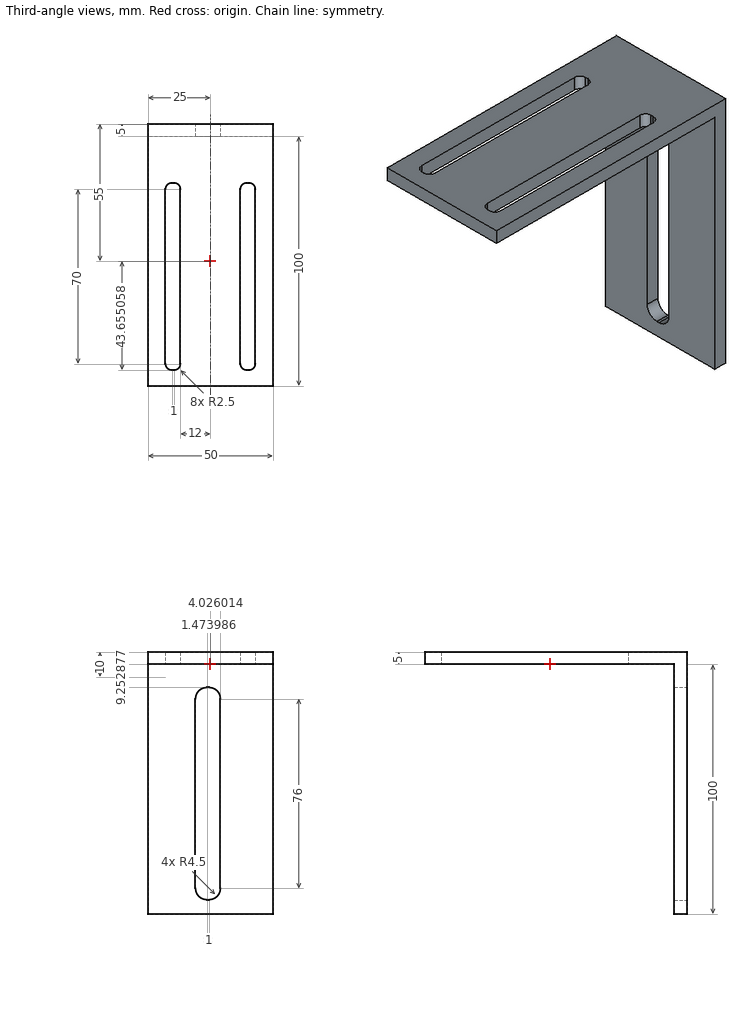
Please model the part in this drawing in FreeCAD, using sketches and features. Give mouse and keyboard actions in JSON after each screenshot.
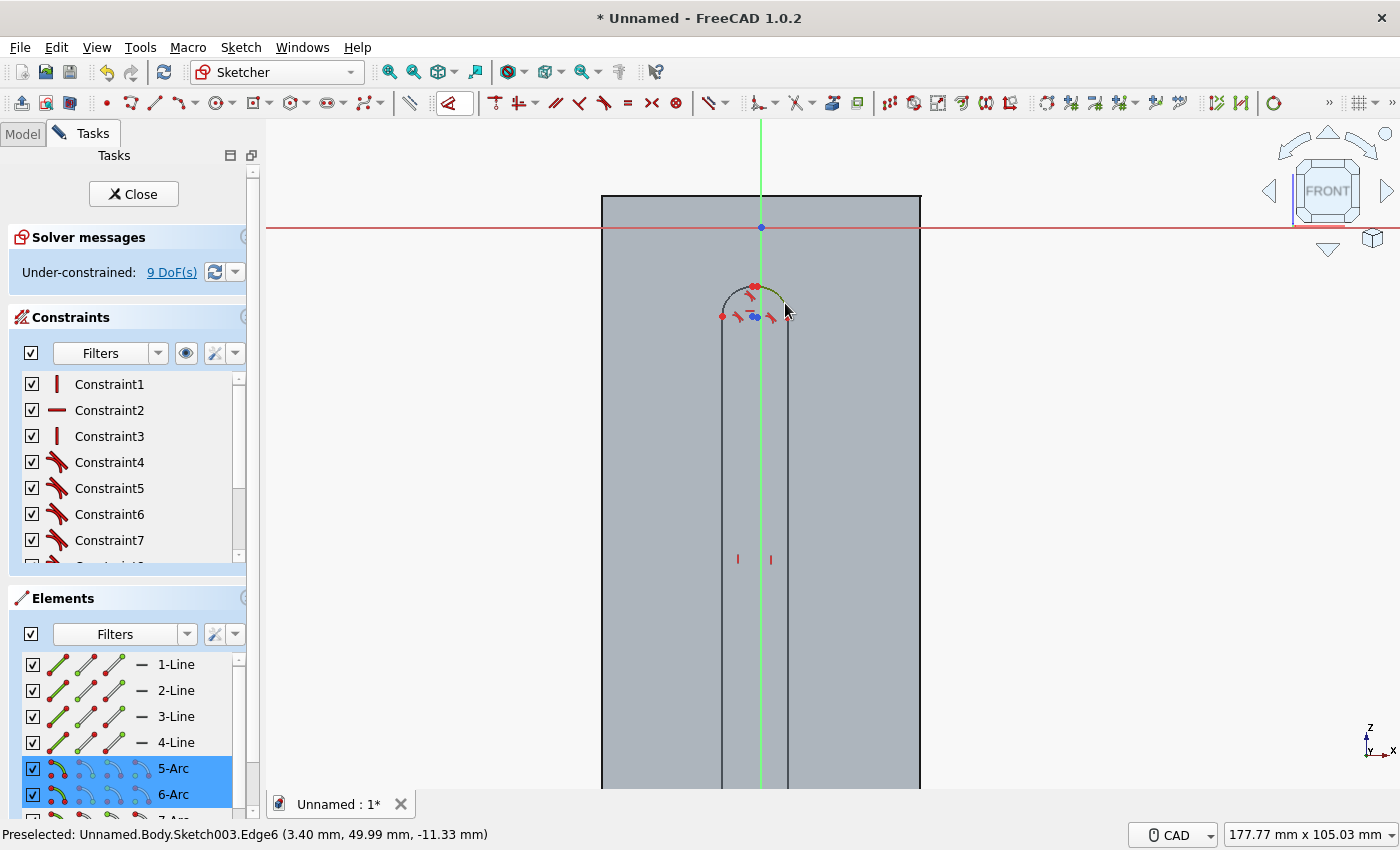
{"action": "left_click", "coordinate": [739, 290]}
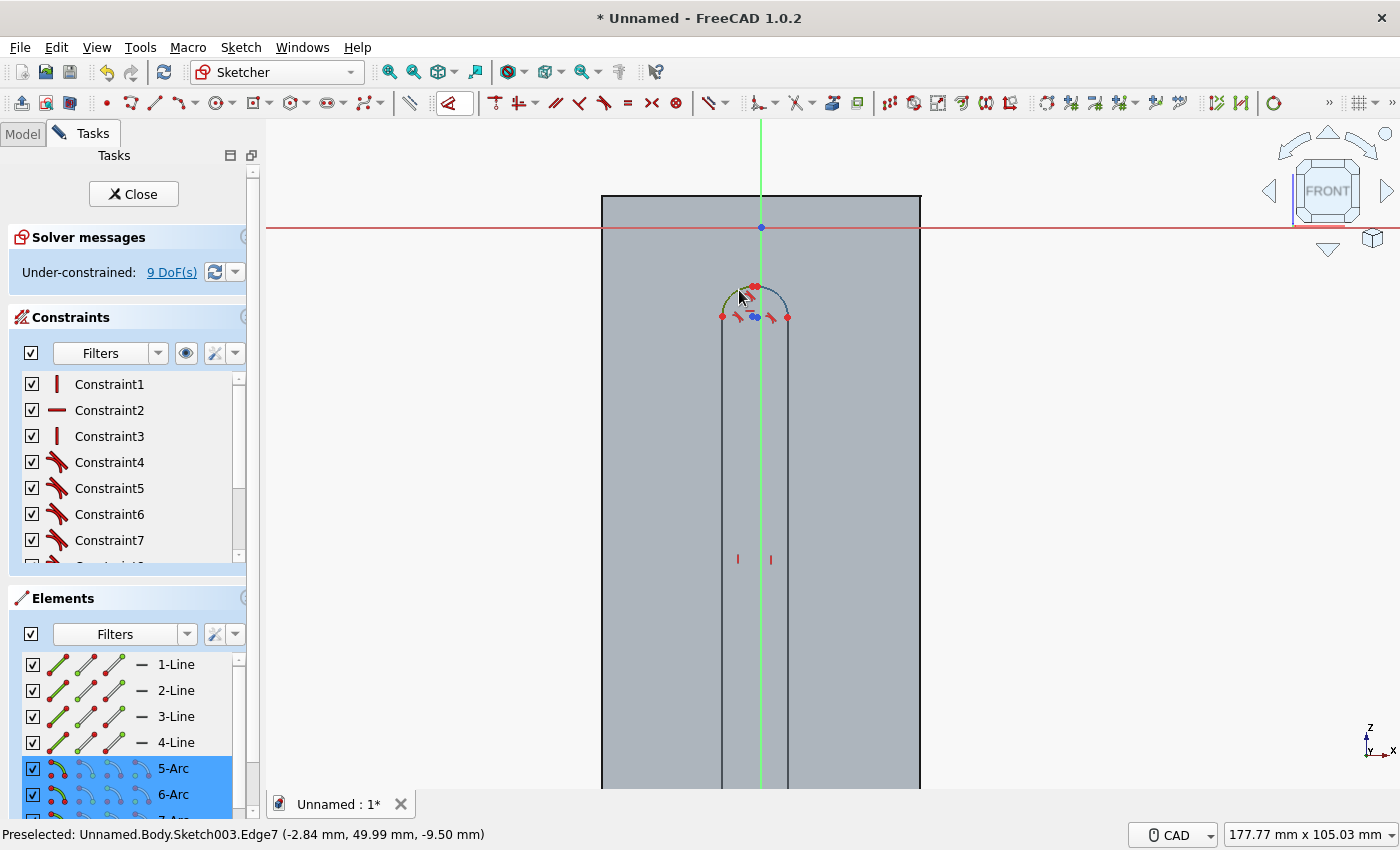
{"action": "scroll", "coordinate": [784, 303], "scroll_direction": "down", "scroll_amount": 2}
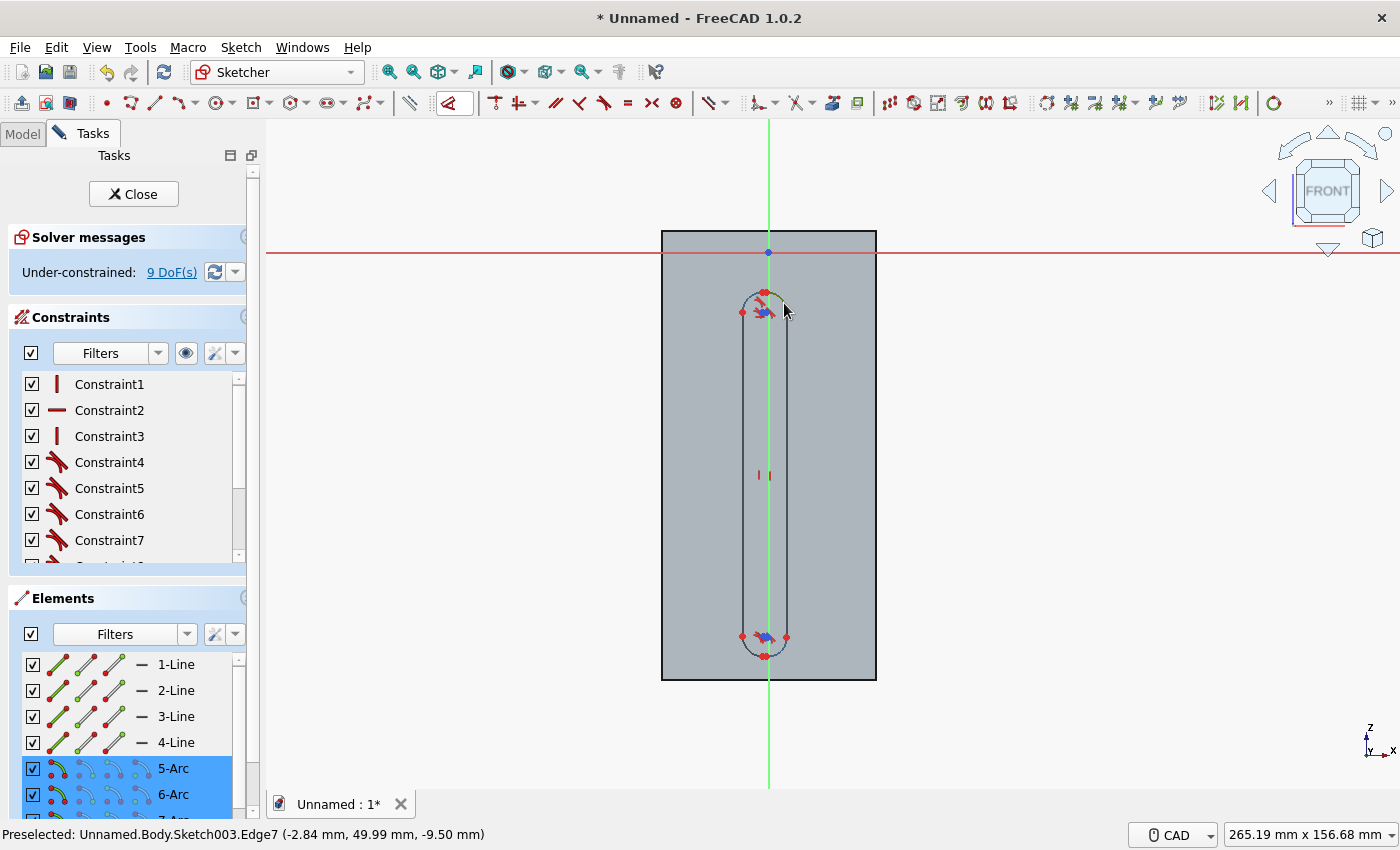
{"action": "scroll", "coordinate": [745, 645], "scroll_direction": "up", "scroll_amount": 2}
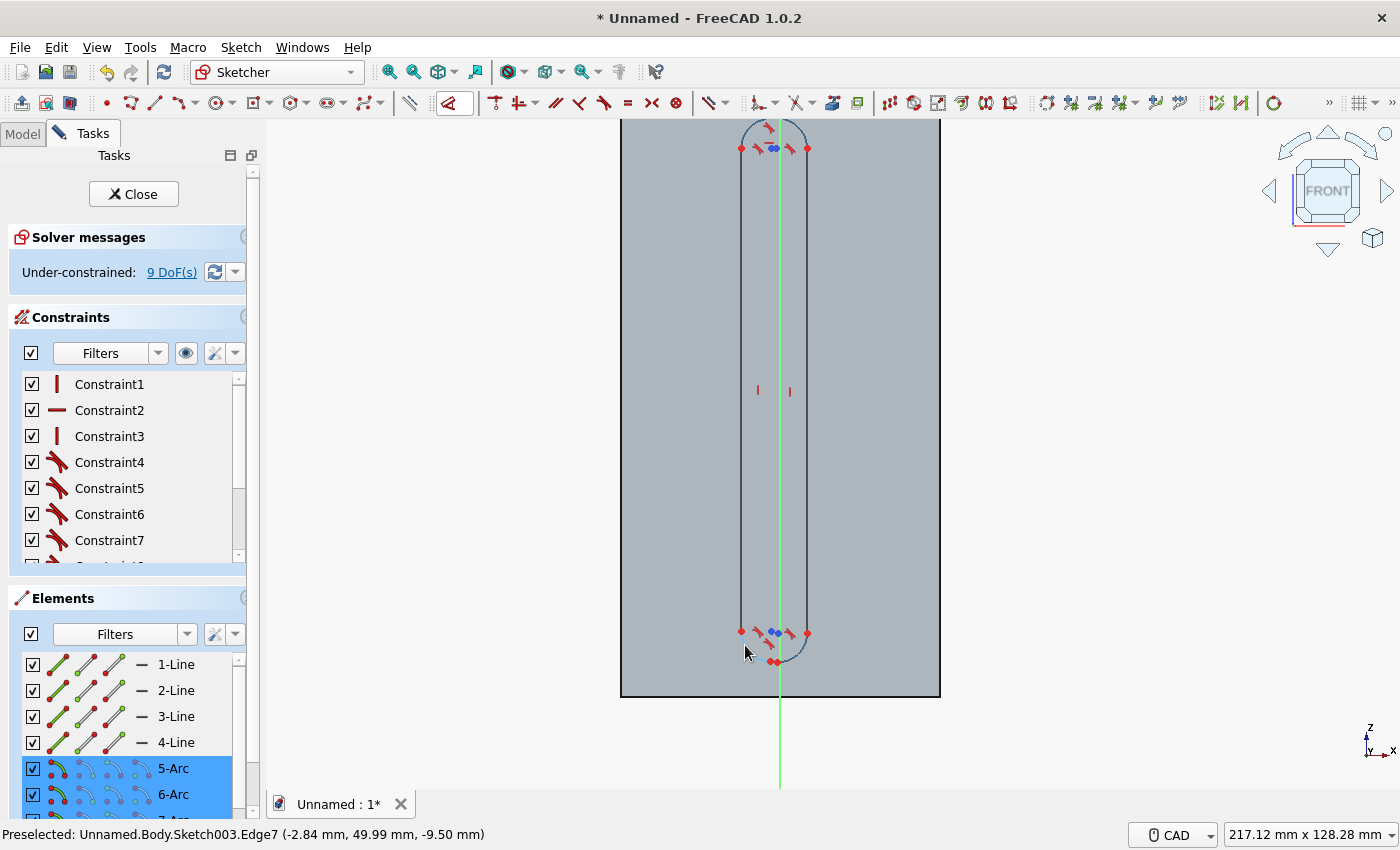
{"action": "left_click", "coordinate": [745, 645]}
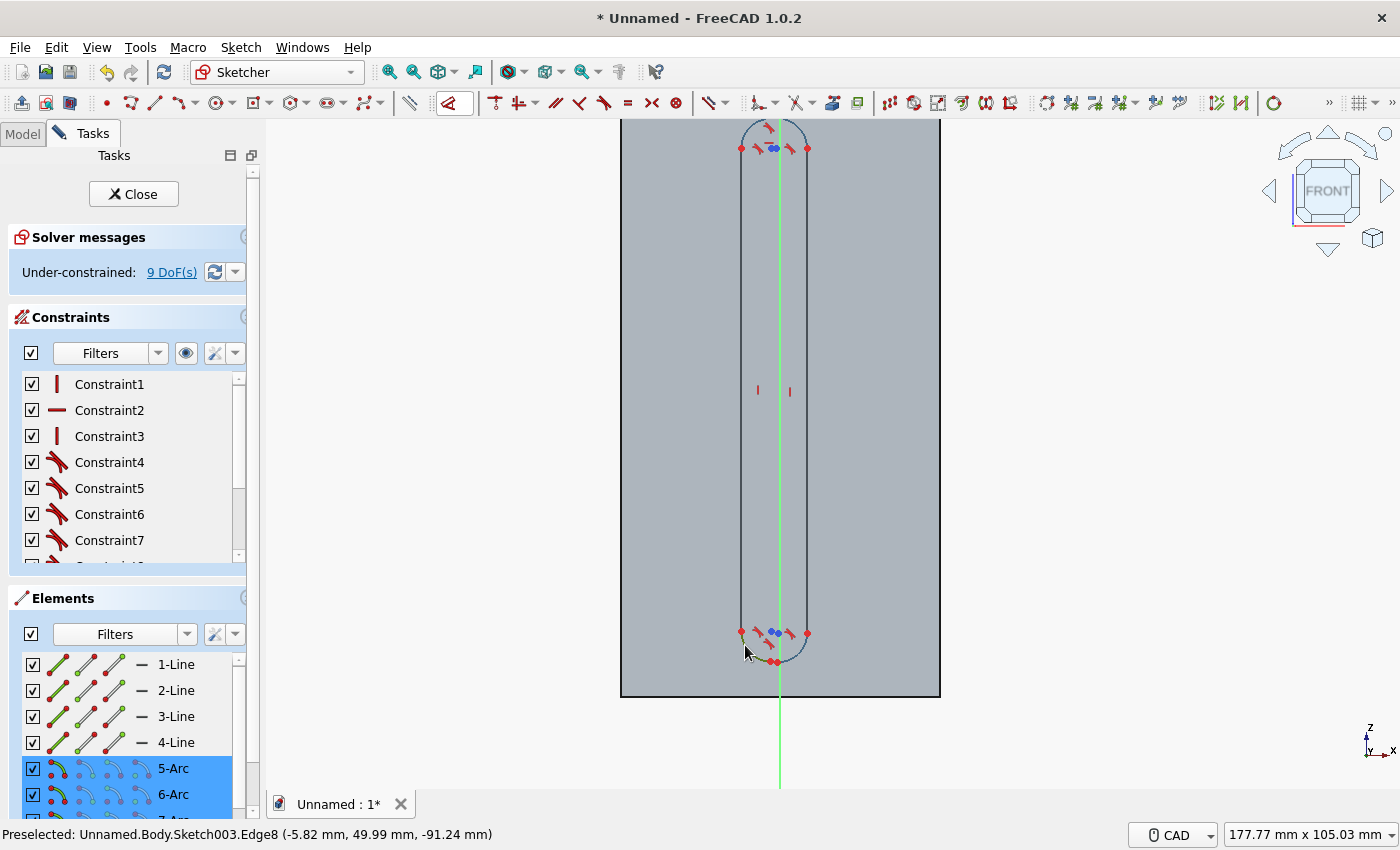
{"action": "key", "text": "e"}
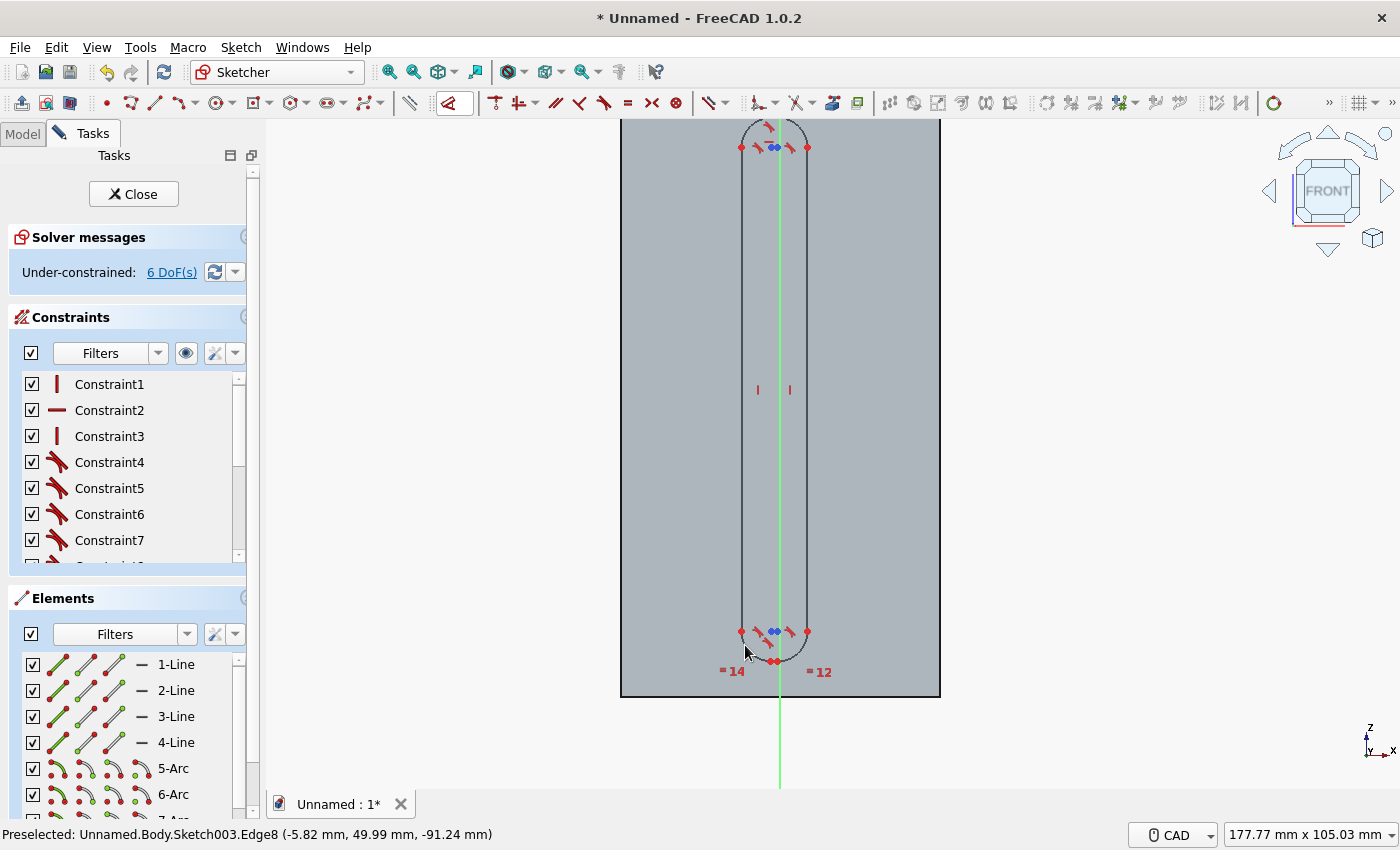
{"action": "scroll", "coordinate": [791, 658], "scroll_direction": "up", "scroll_amount": 2}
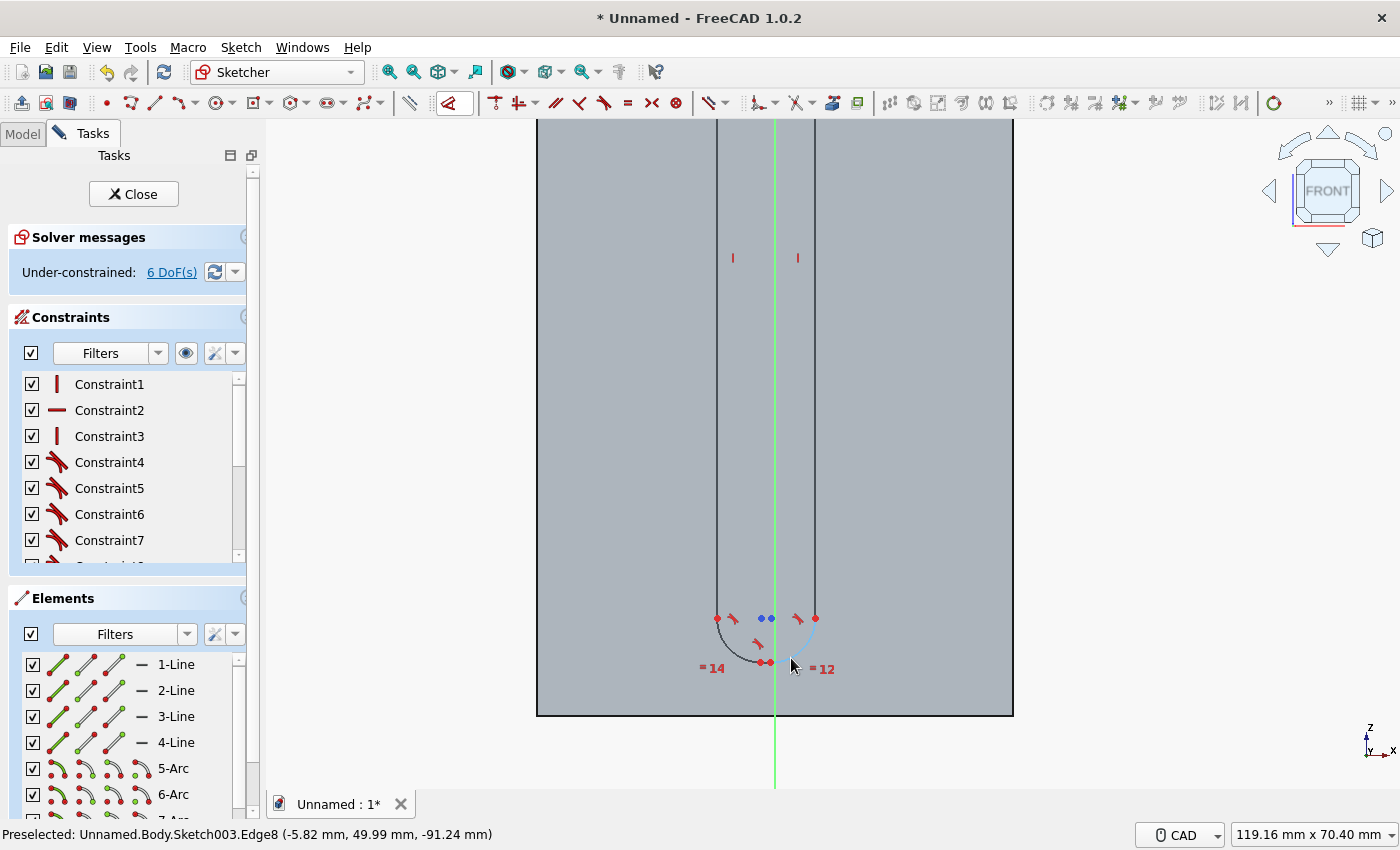
{"action": "left_click", "coordinate": [791, 658]}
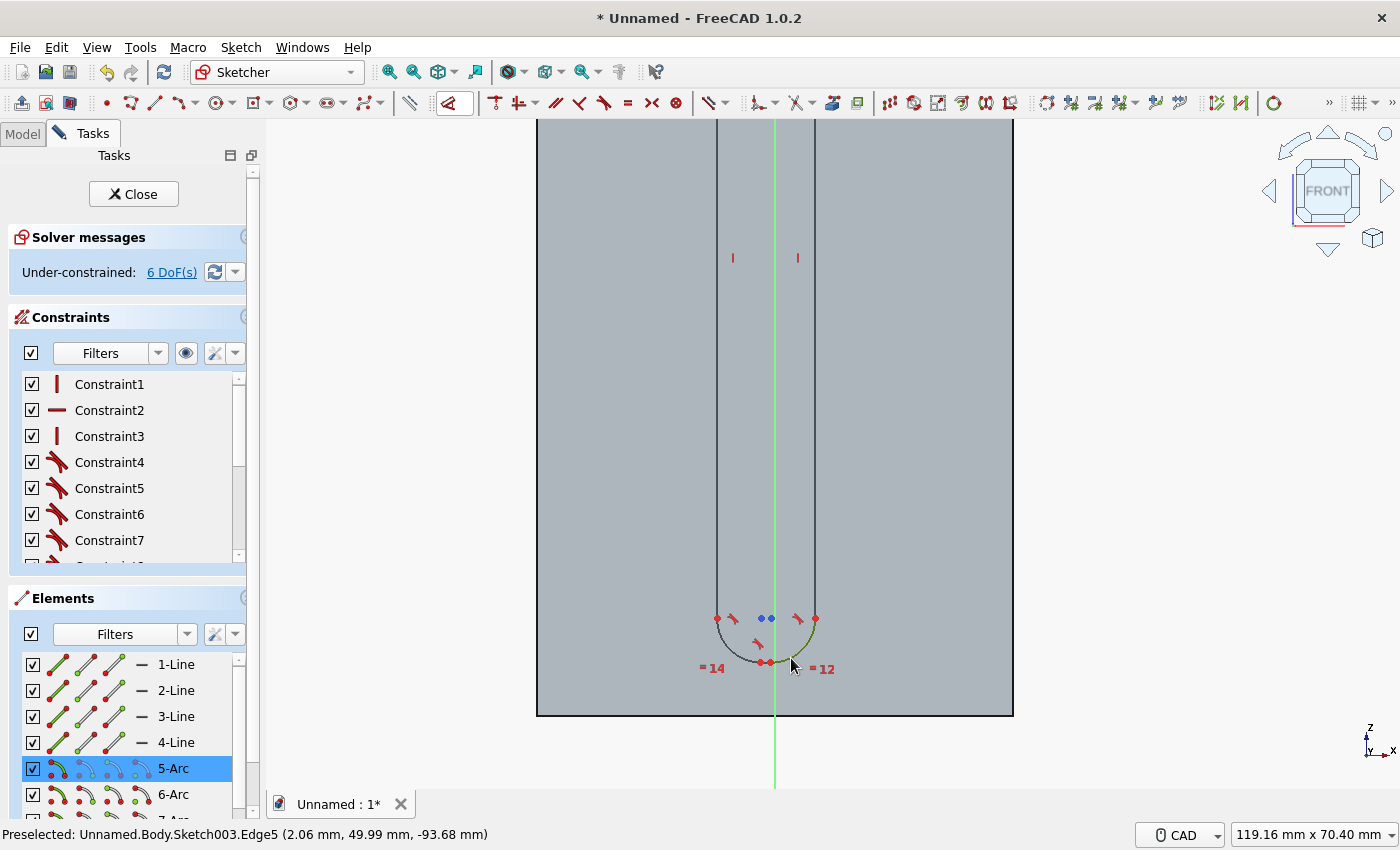
{"action": "key", "text": "k r"}